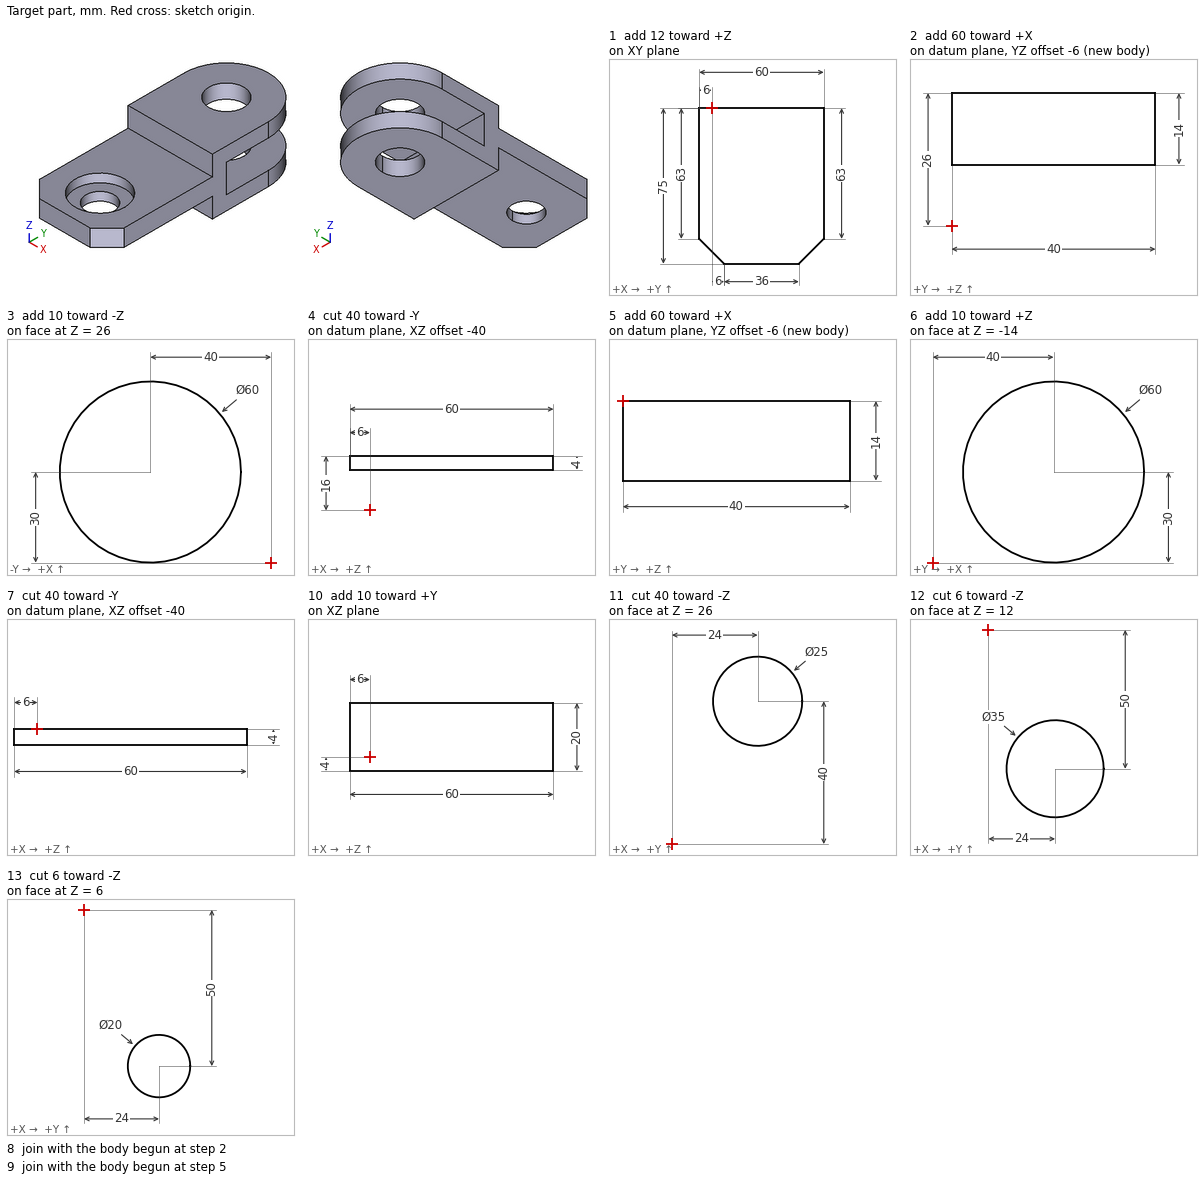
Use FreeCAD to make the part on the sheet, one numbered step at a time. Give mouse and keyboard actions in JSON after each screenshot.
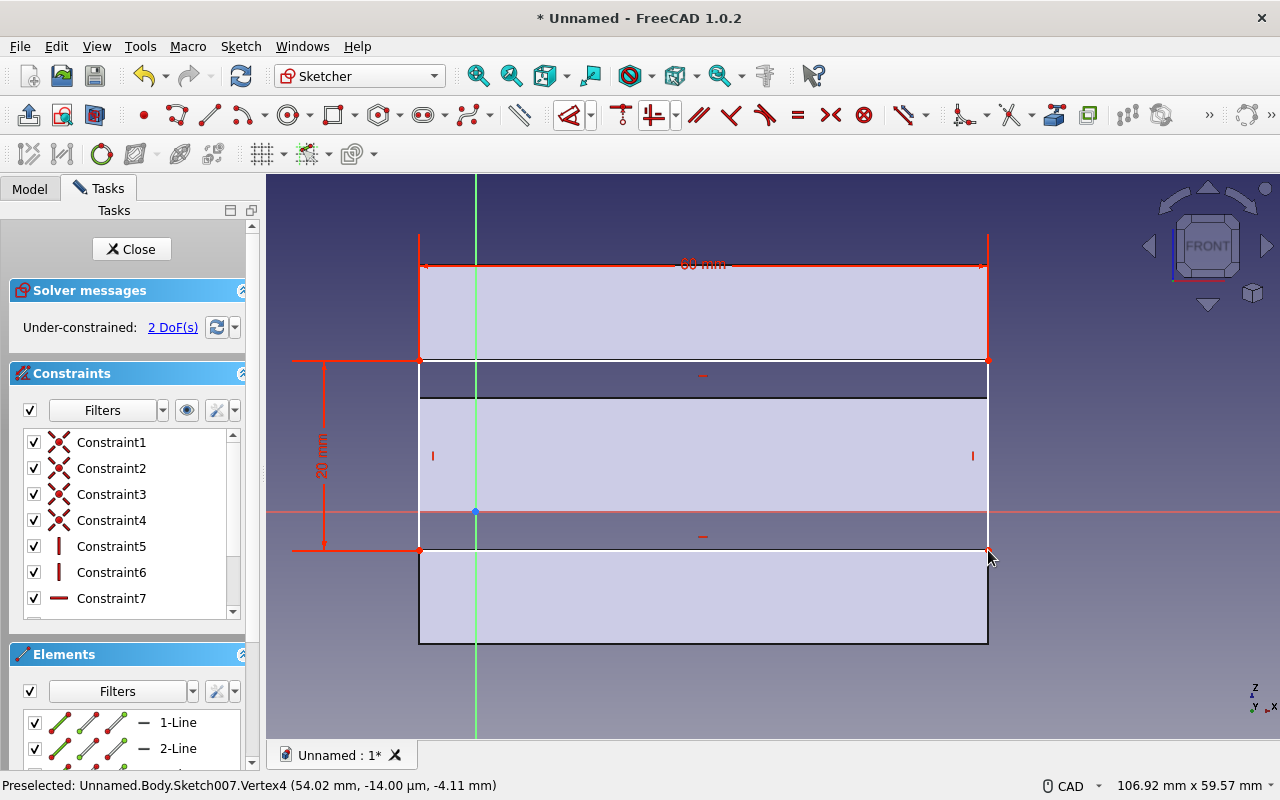
{"action": "left_click", "coordinate": [419, 361]}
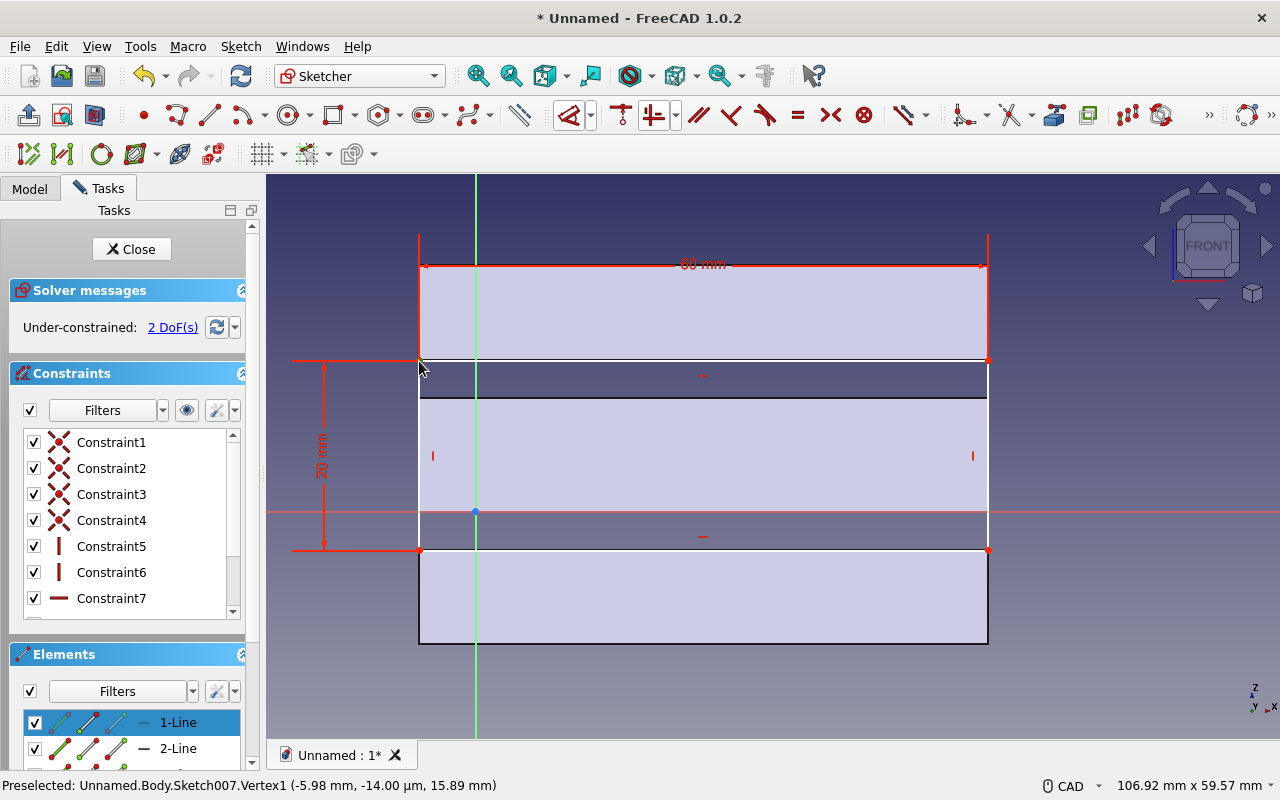
{"action": "left_click", "coordinate": [590, 116]}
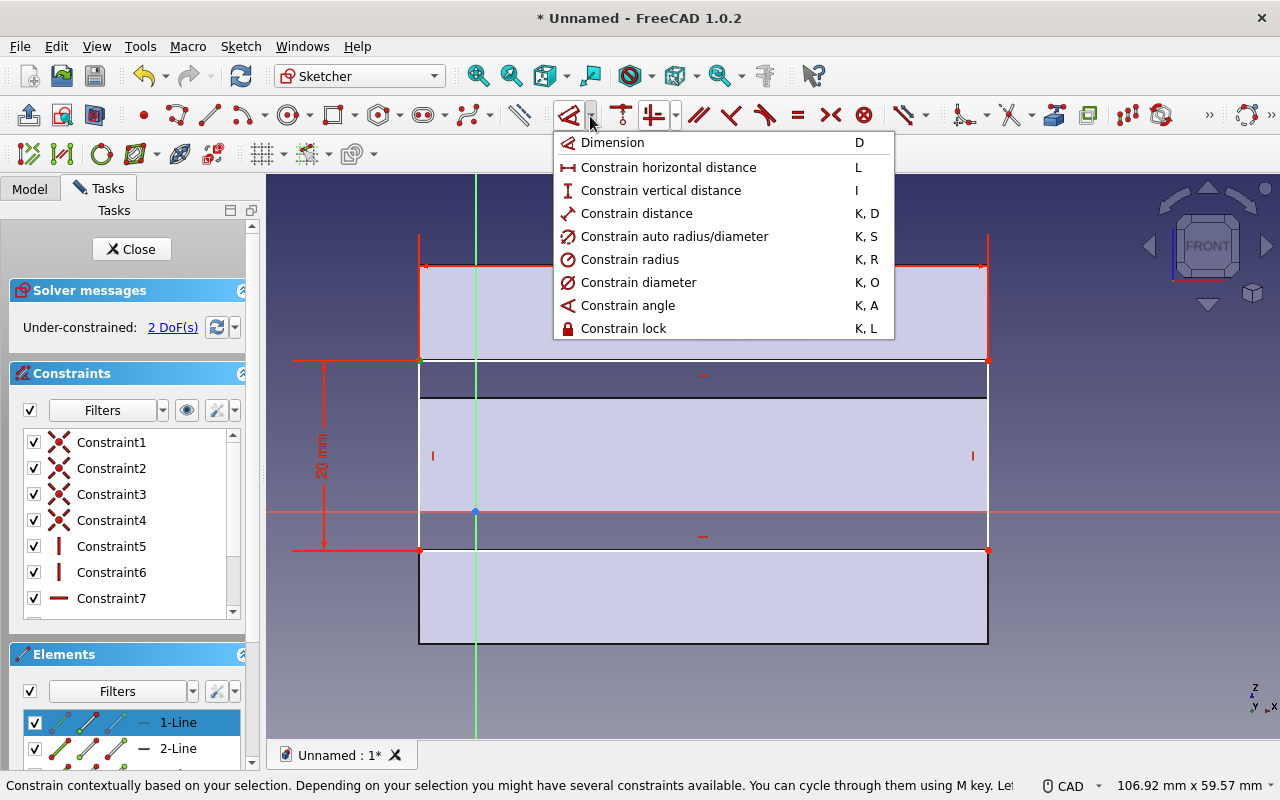
{"action": "left_click", "coordinate": [724, 168]}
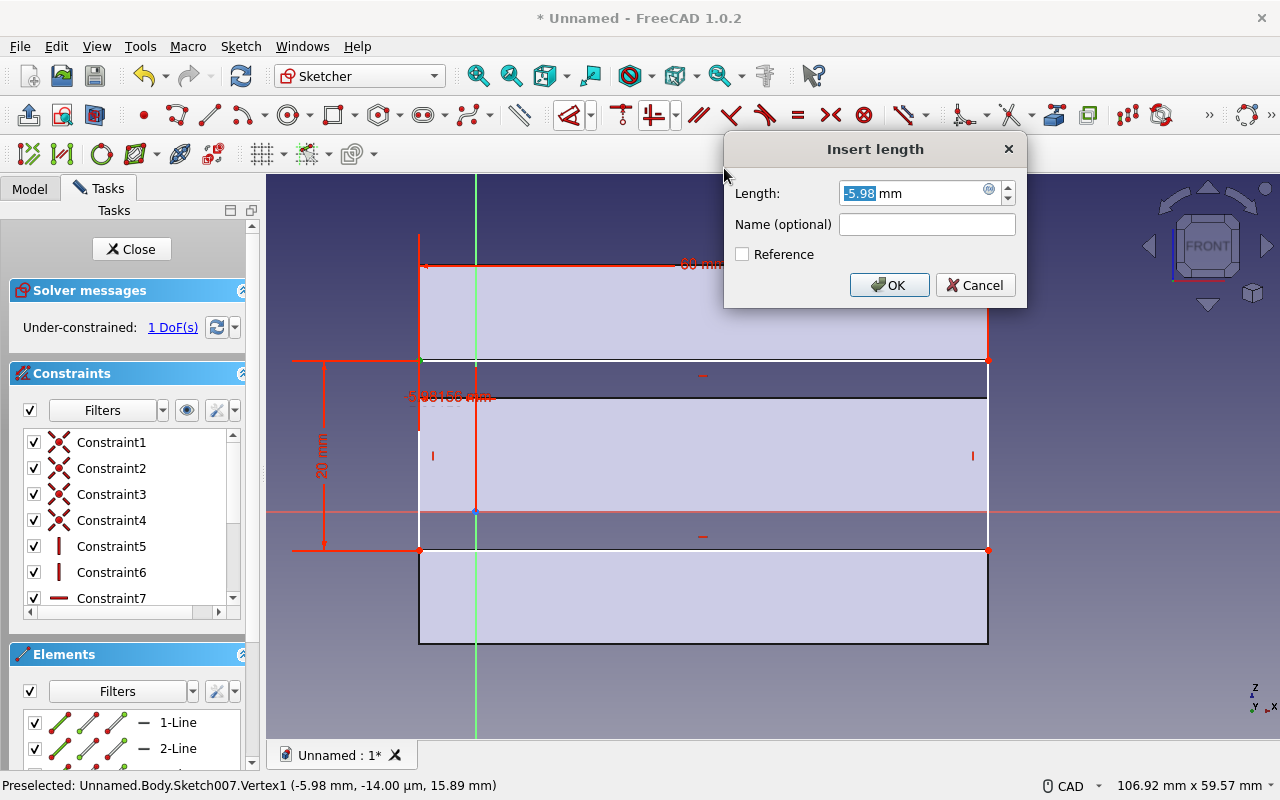
{"action": "type", "text": "-6"}
{"action": "key", "text": "Return"}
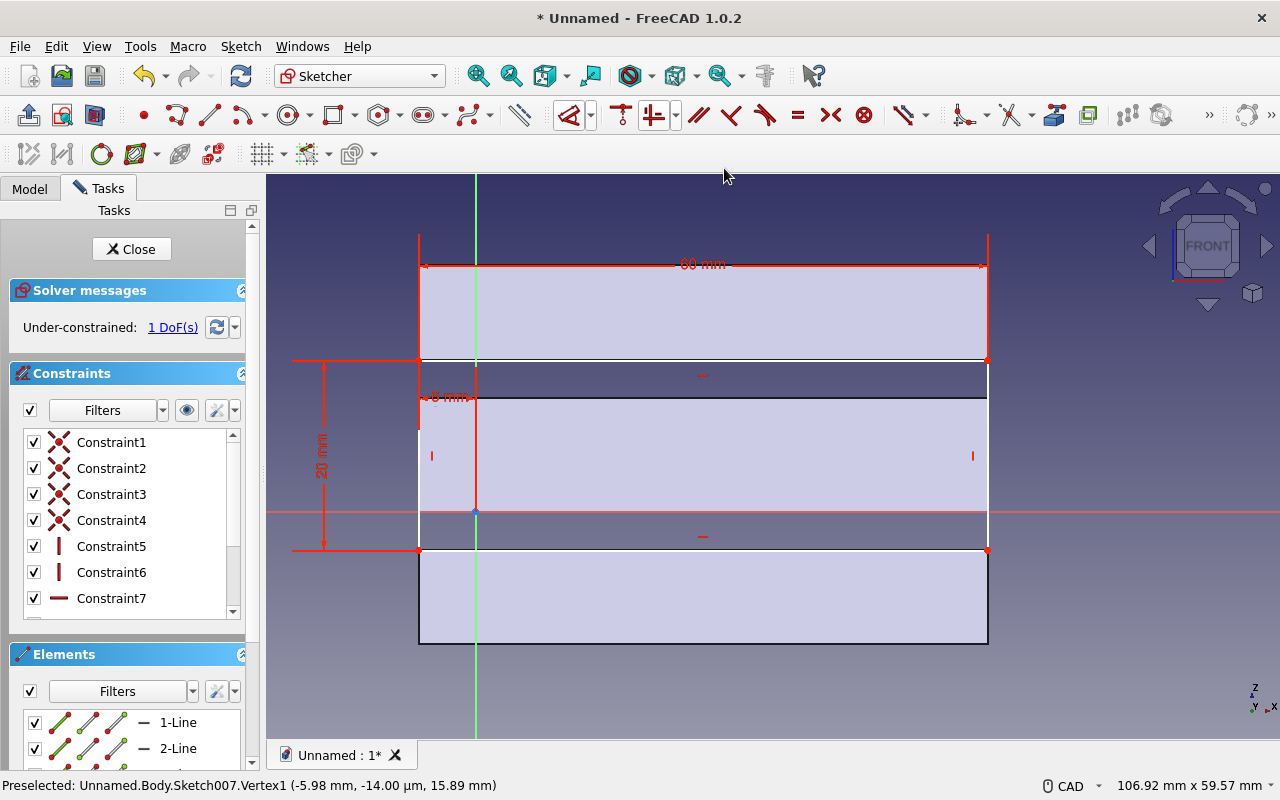
{"action": "left_click", "coordinate": [419, 551]}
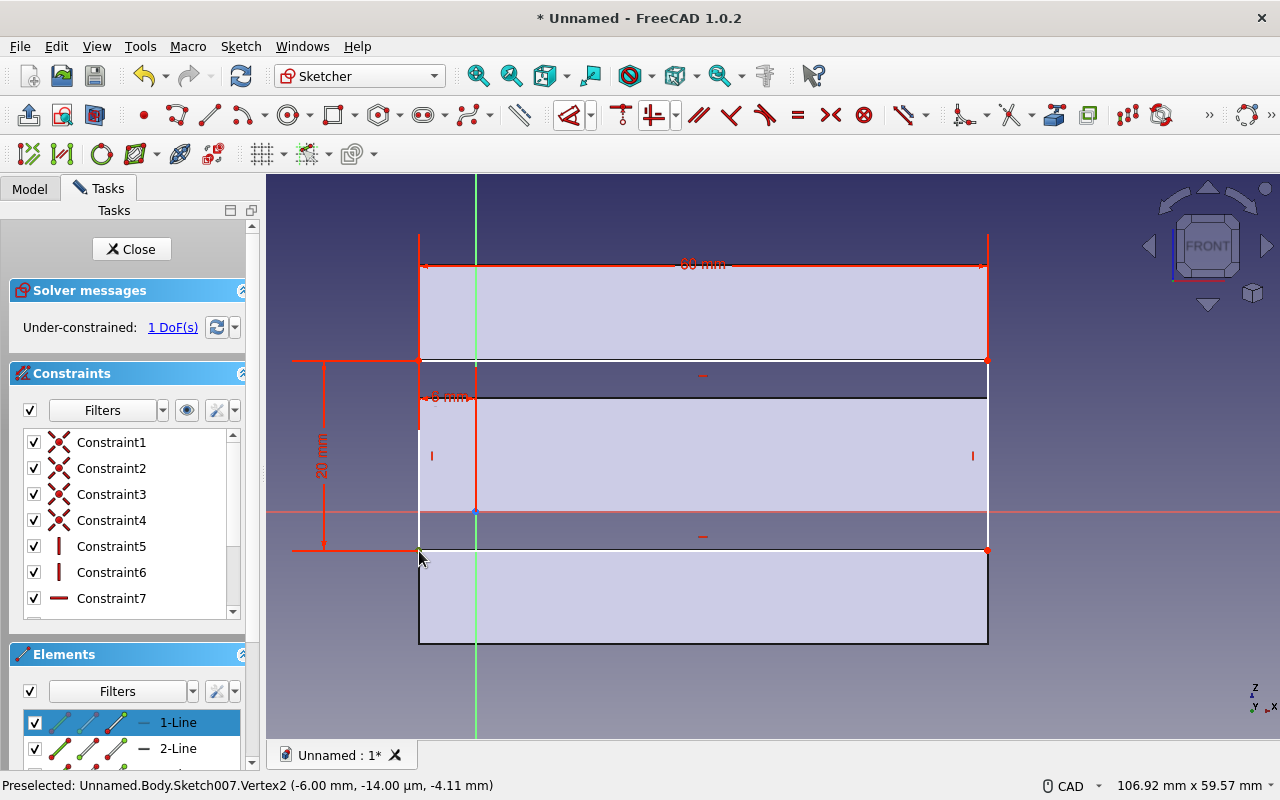
{"action": "key", "text": "i"}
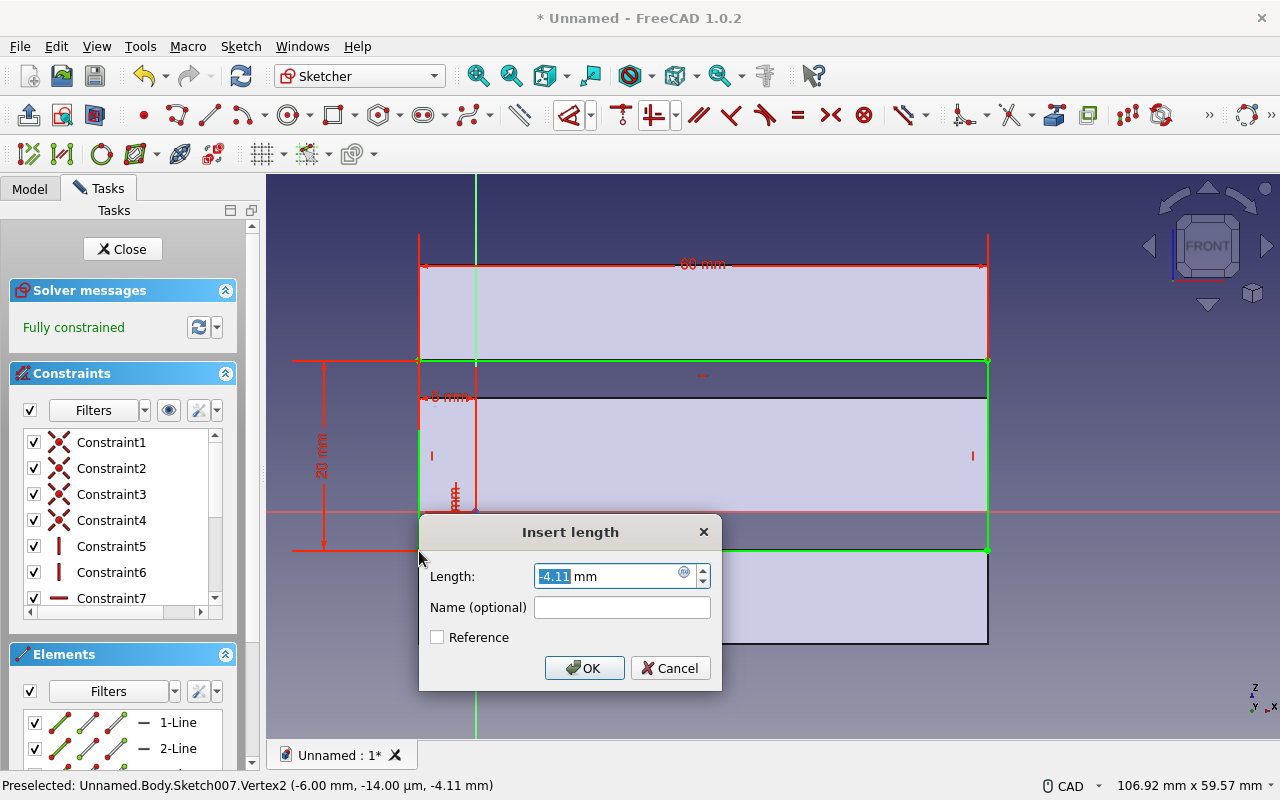
{"action": "type", "text": "-4"}
{"action": "key", "text": "Return"}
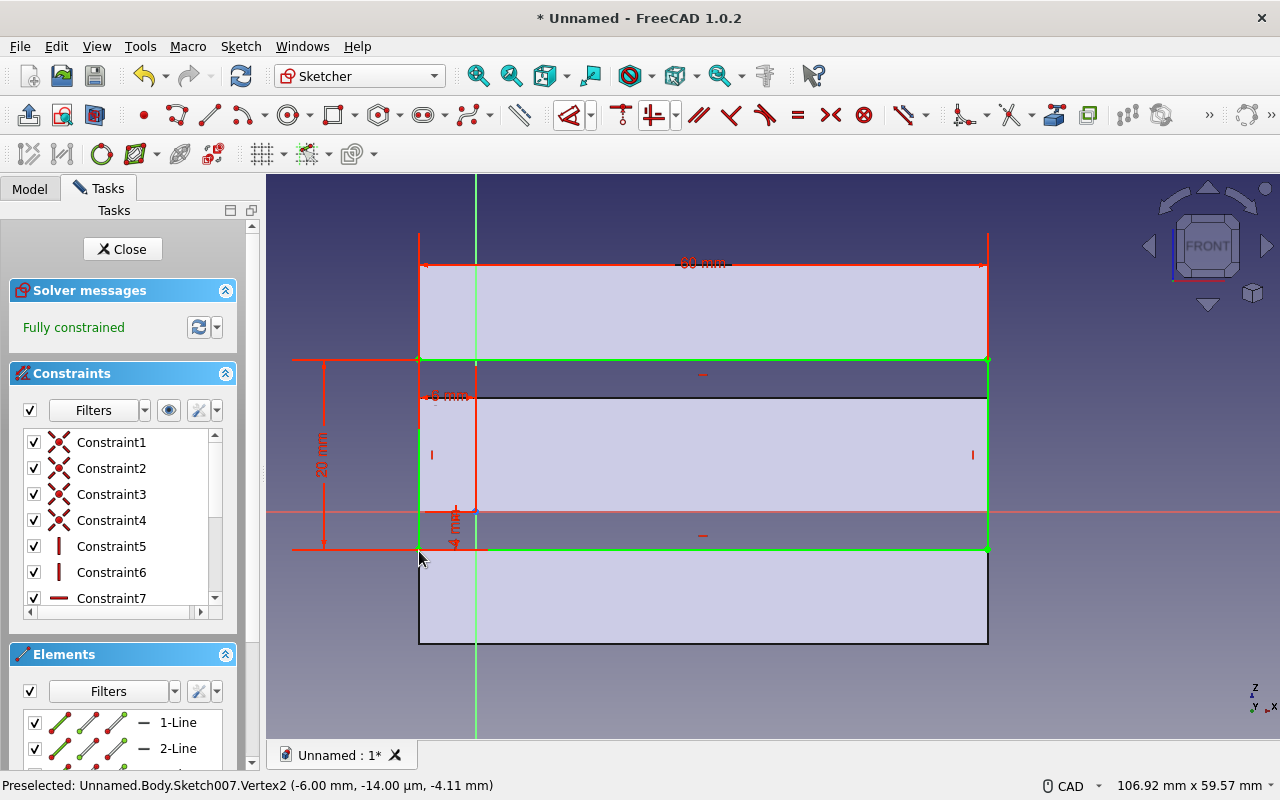
{"action": "left_click", "coordinate": [123, 249]}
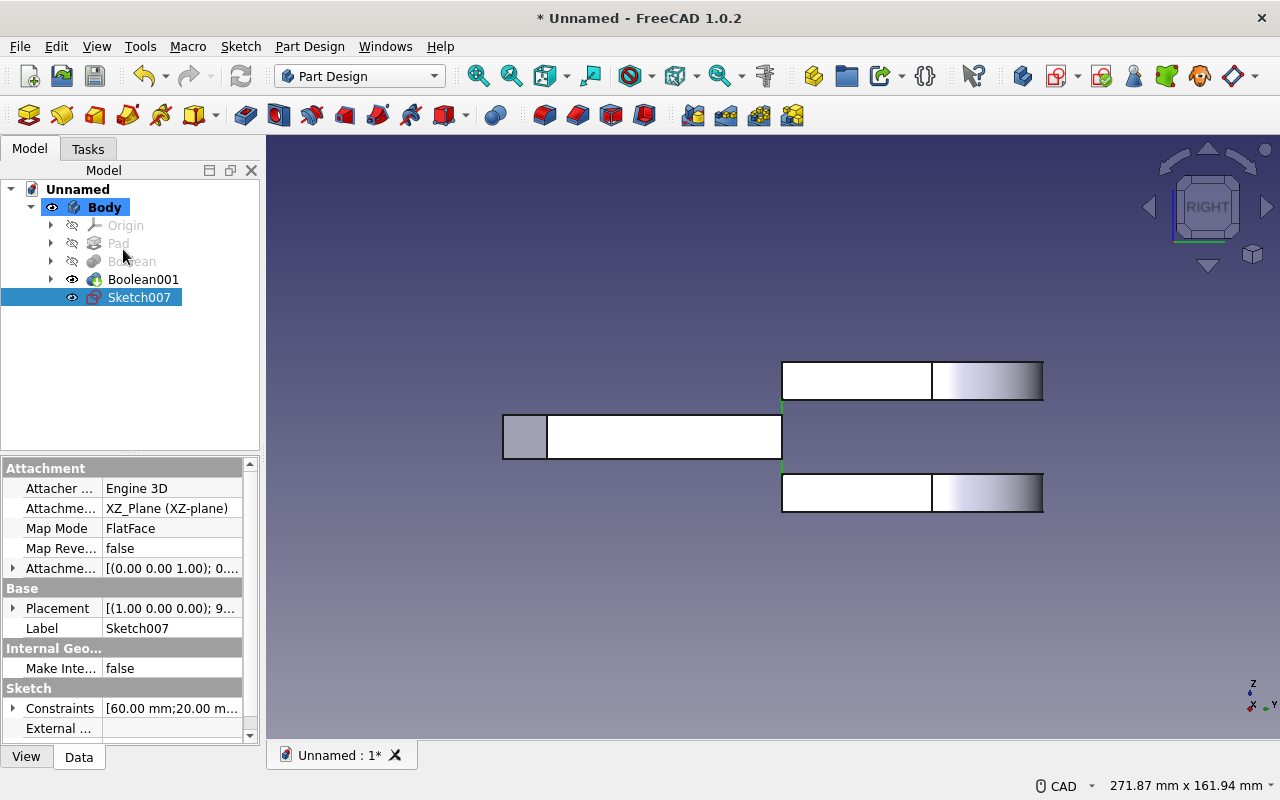
{"action": "left_click", "coordinate": [29, 116]}